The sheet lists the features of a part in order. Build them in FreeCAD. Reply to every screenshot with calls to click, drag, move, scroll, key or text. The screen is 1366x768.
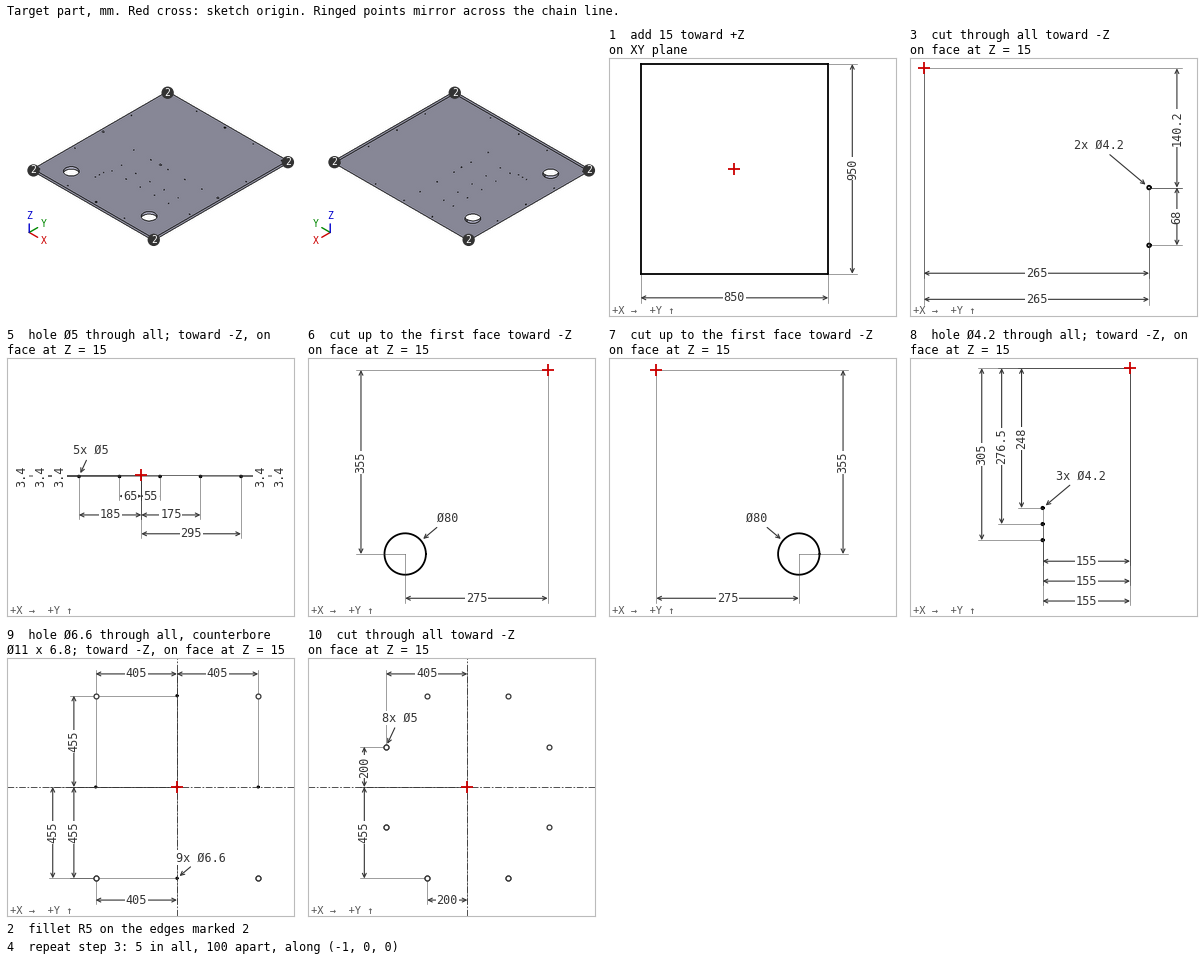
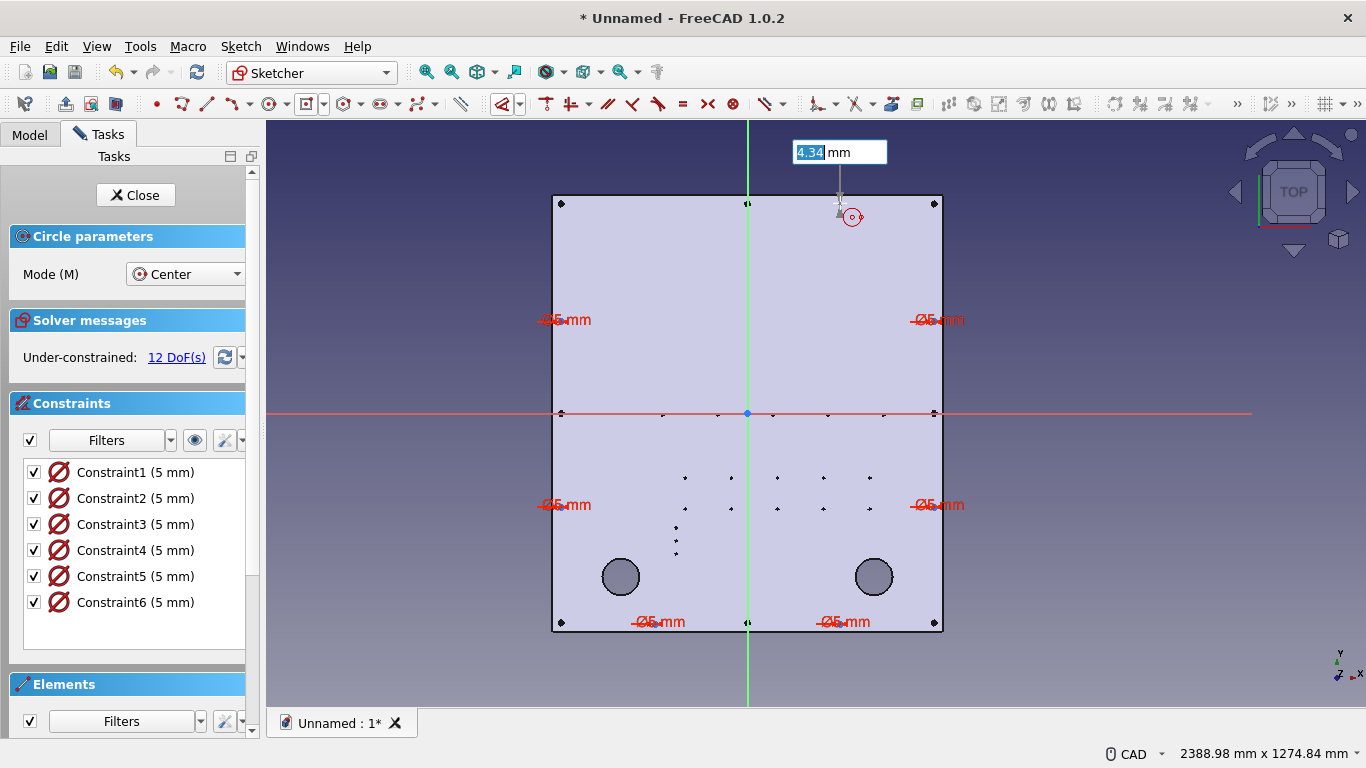
text(5)
key(Return)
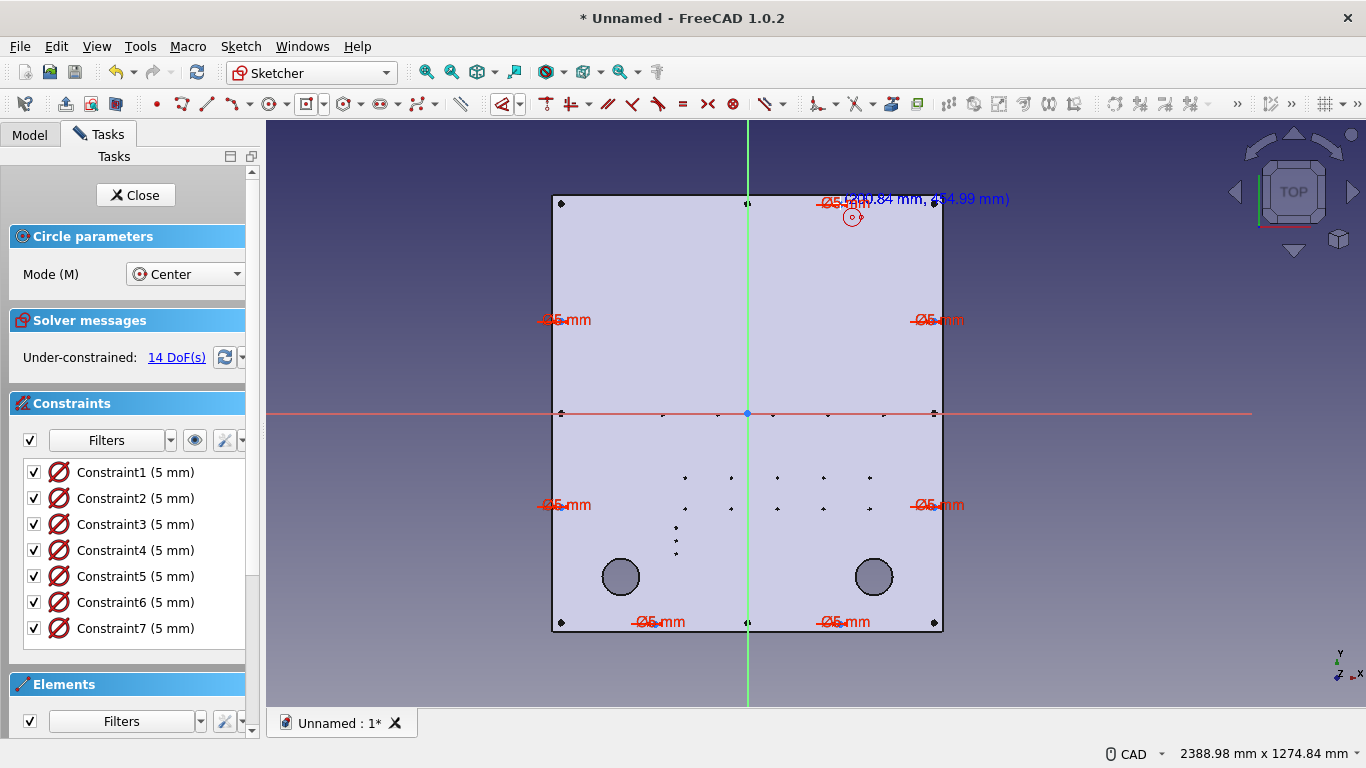
scroll(655, 204, up, 15)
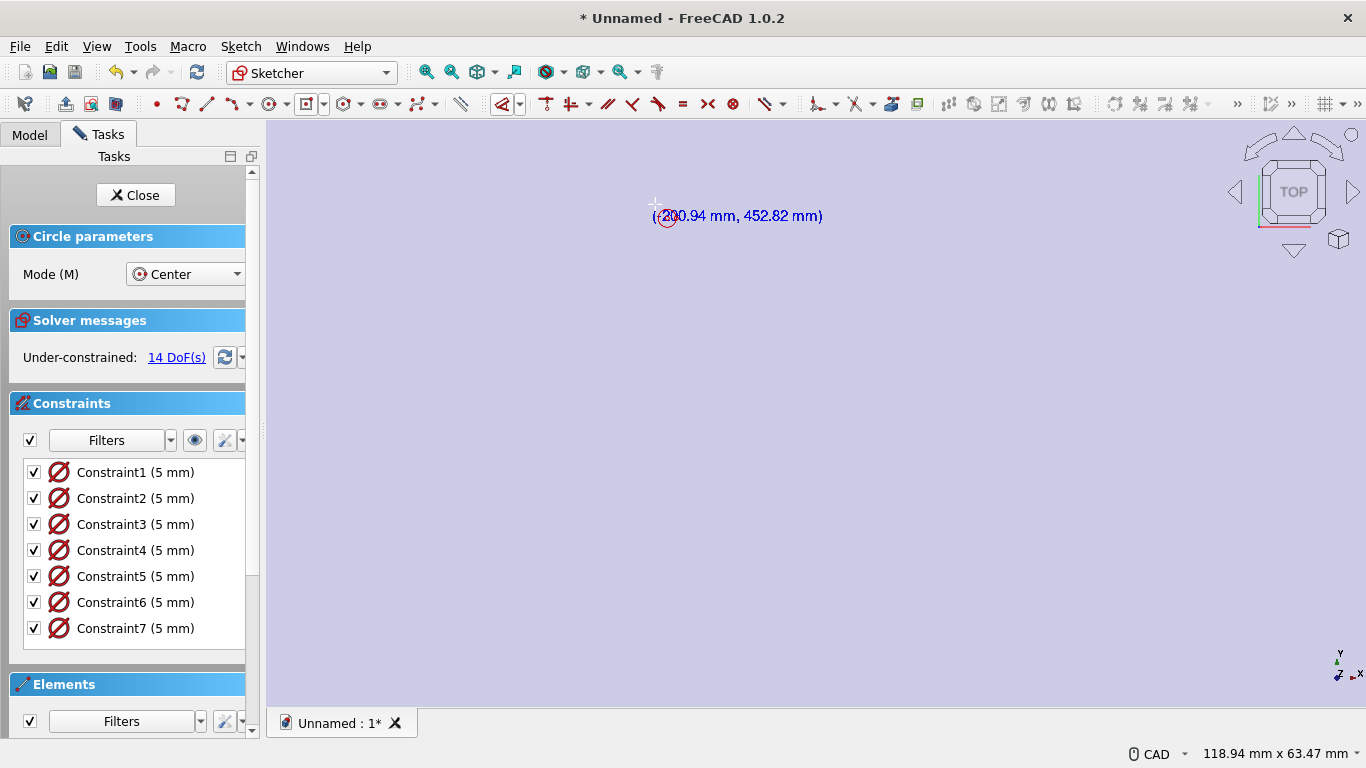
scroll(655, 204, down, 15)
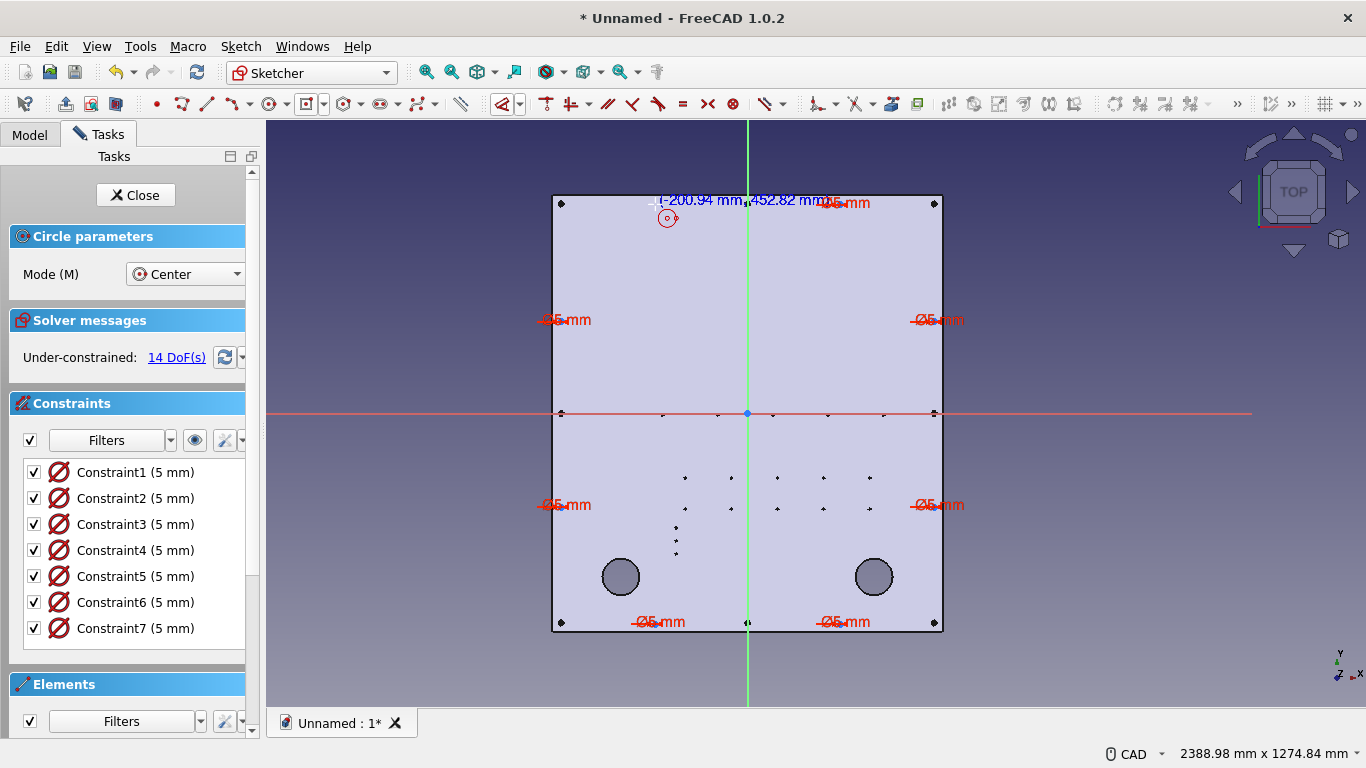
click(655, 204)
move(656, 203)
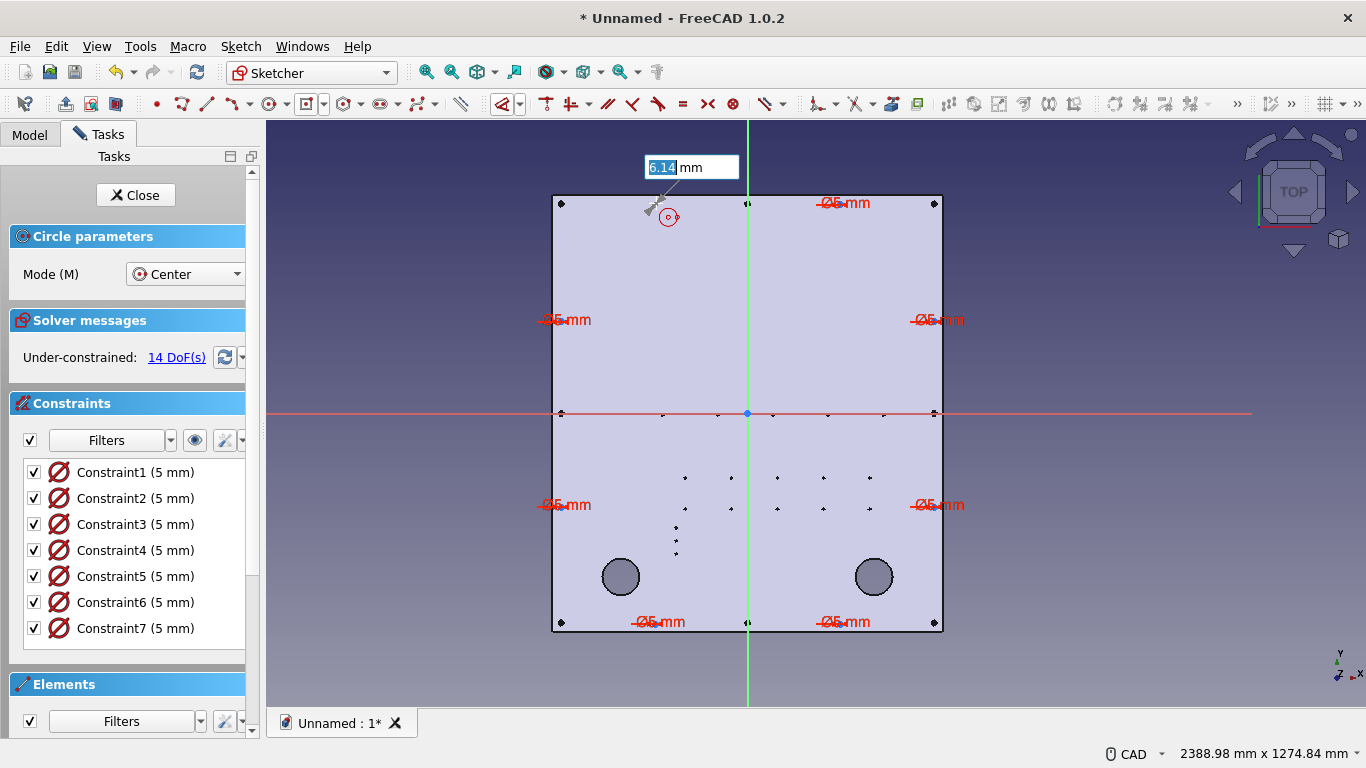
text(5)
key(Return)
key(Escape)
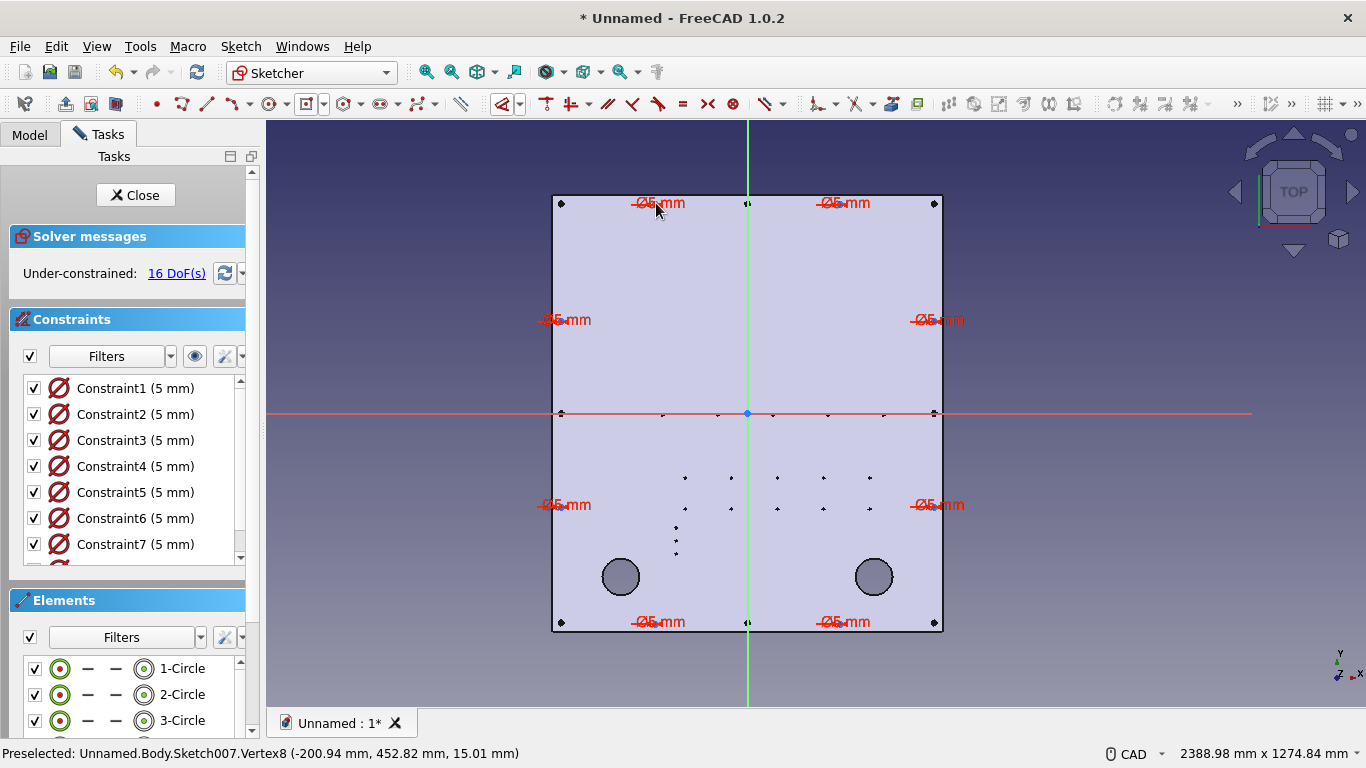
click(561, 322)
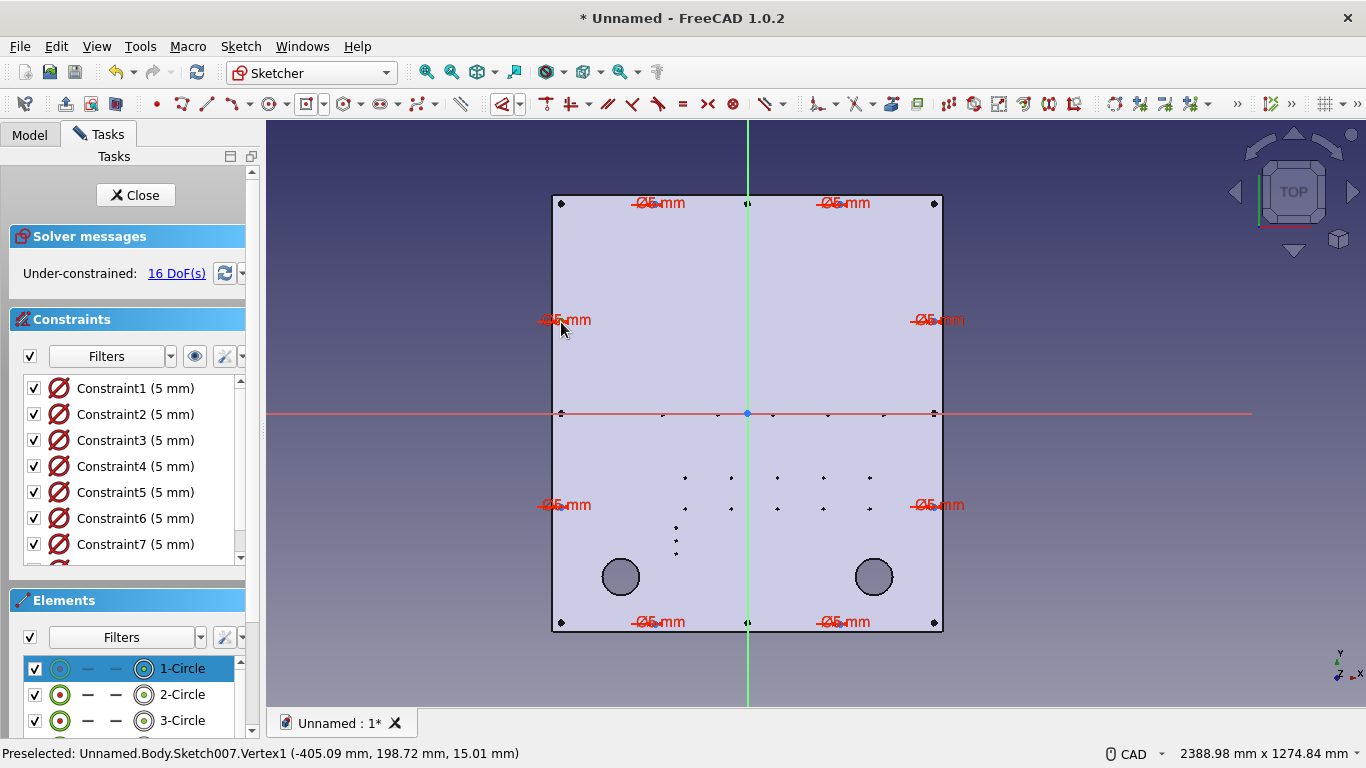
click(561, 507)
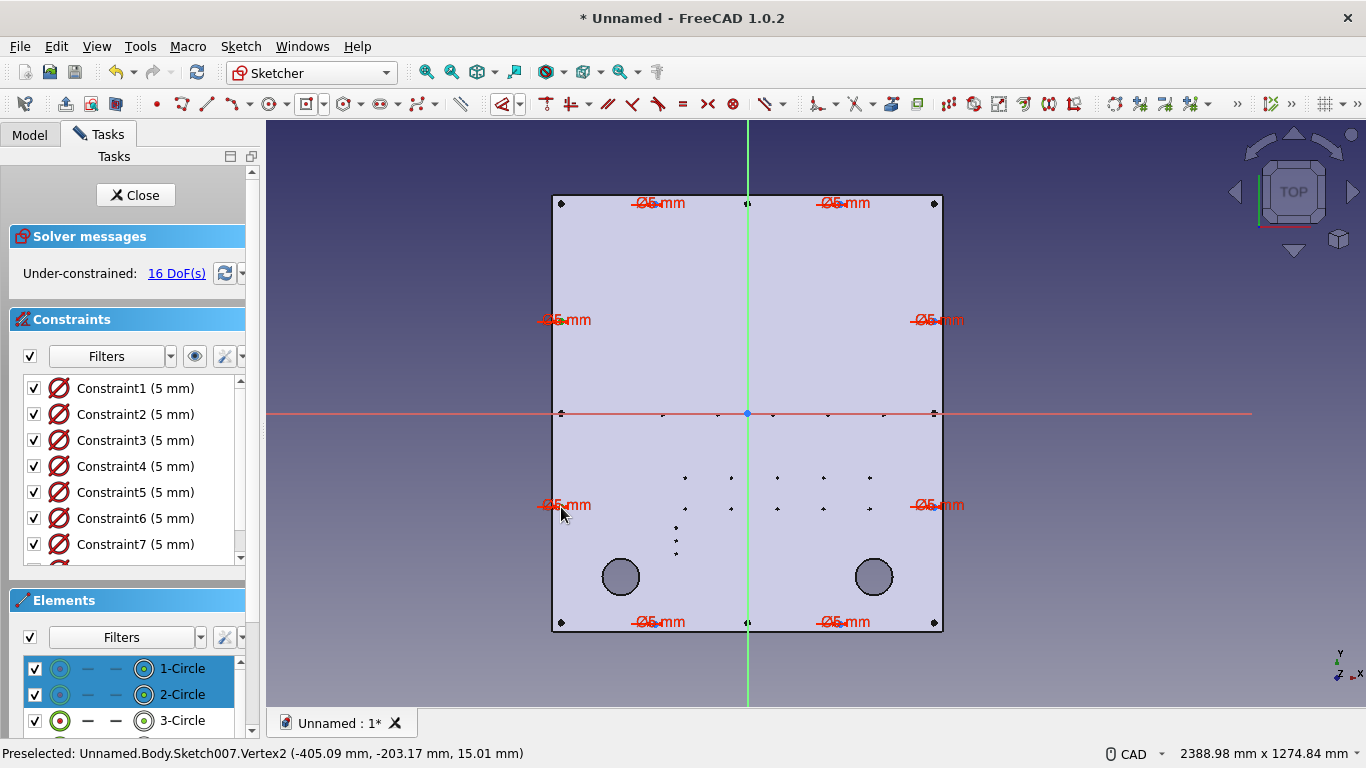
click(359, 413)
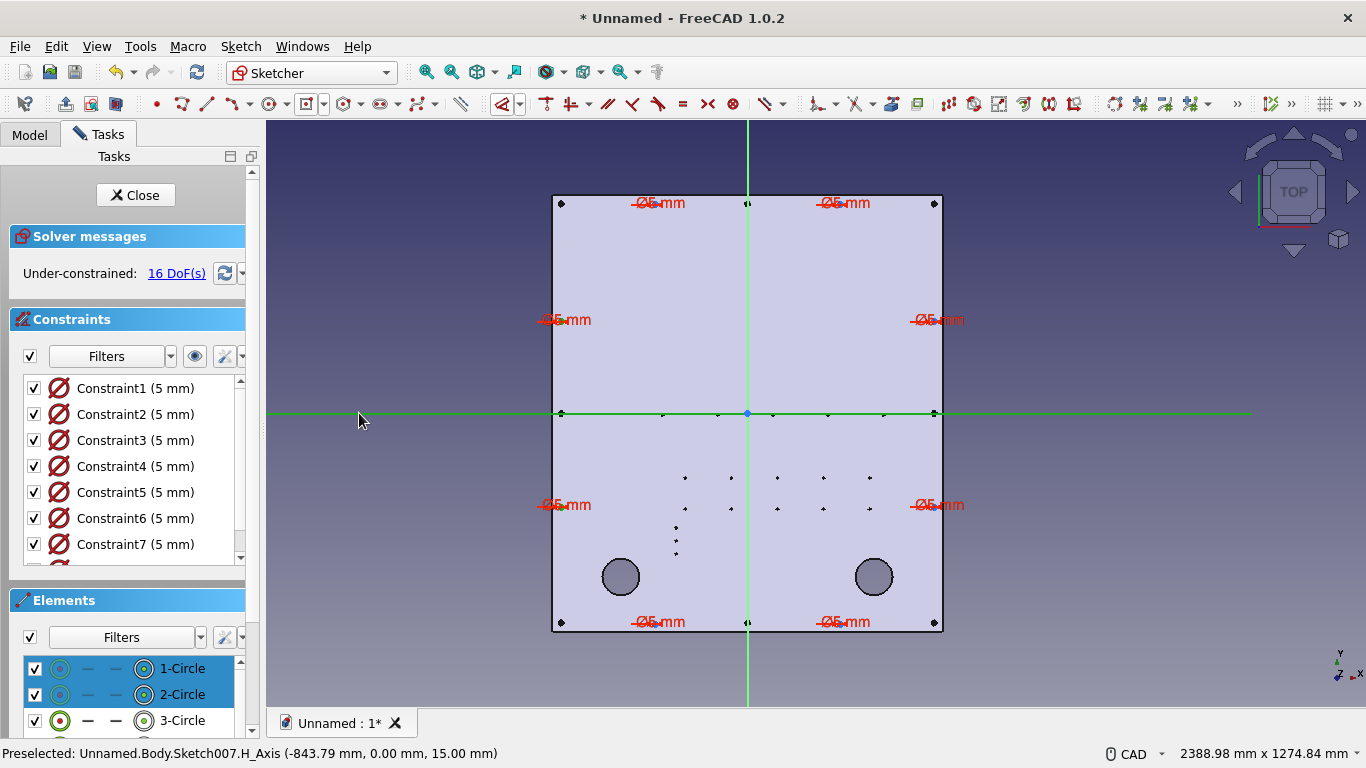
click(708, 104)